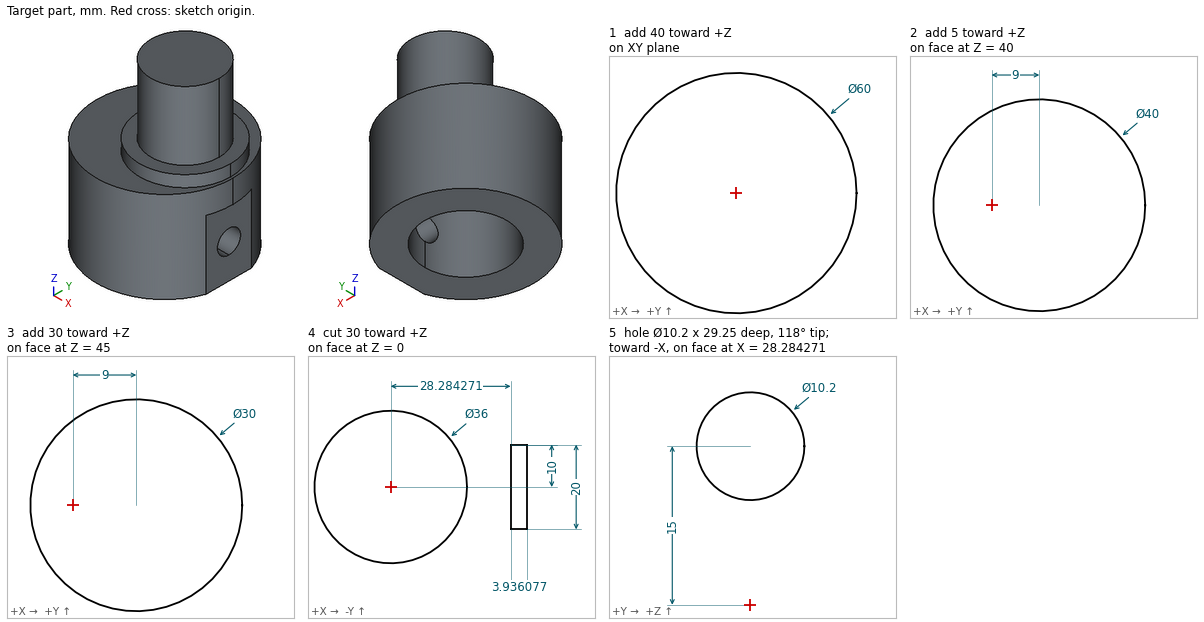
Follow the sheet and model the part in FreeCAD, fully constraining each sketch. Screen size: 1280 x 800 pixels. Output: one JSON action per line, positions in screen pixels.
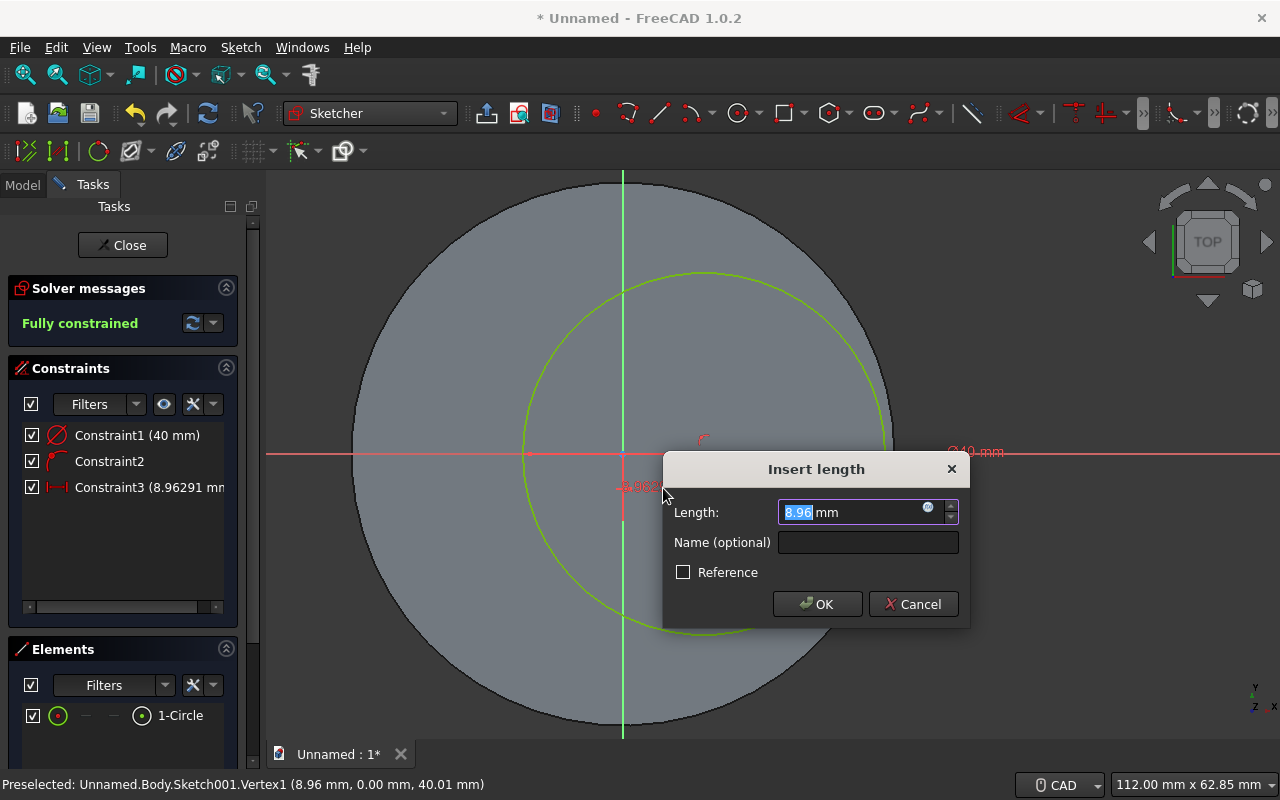
{"action": "type", "text": "9"}
{"action": "key", "text": "Return"}
{"action": "key", "text": "Escape"}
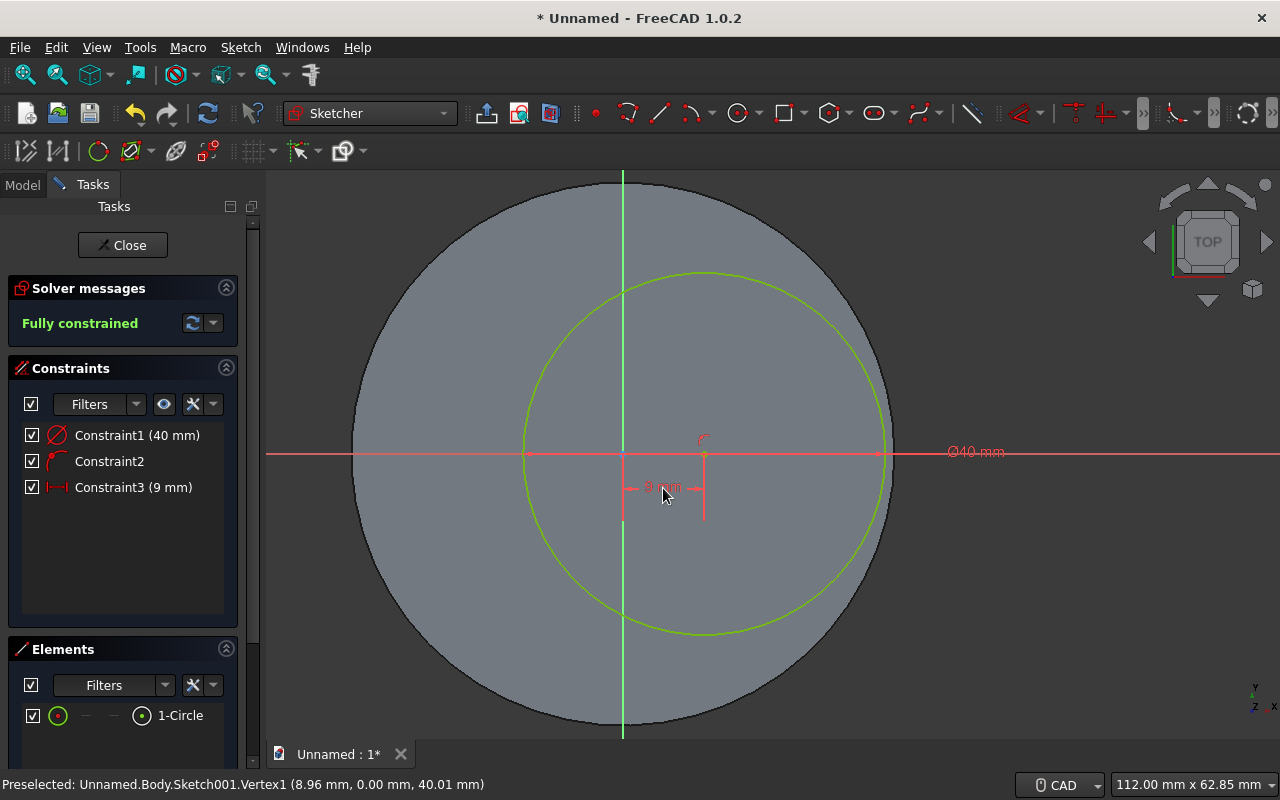
{"action": "left_click", "coordinate": [123, 245]}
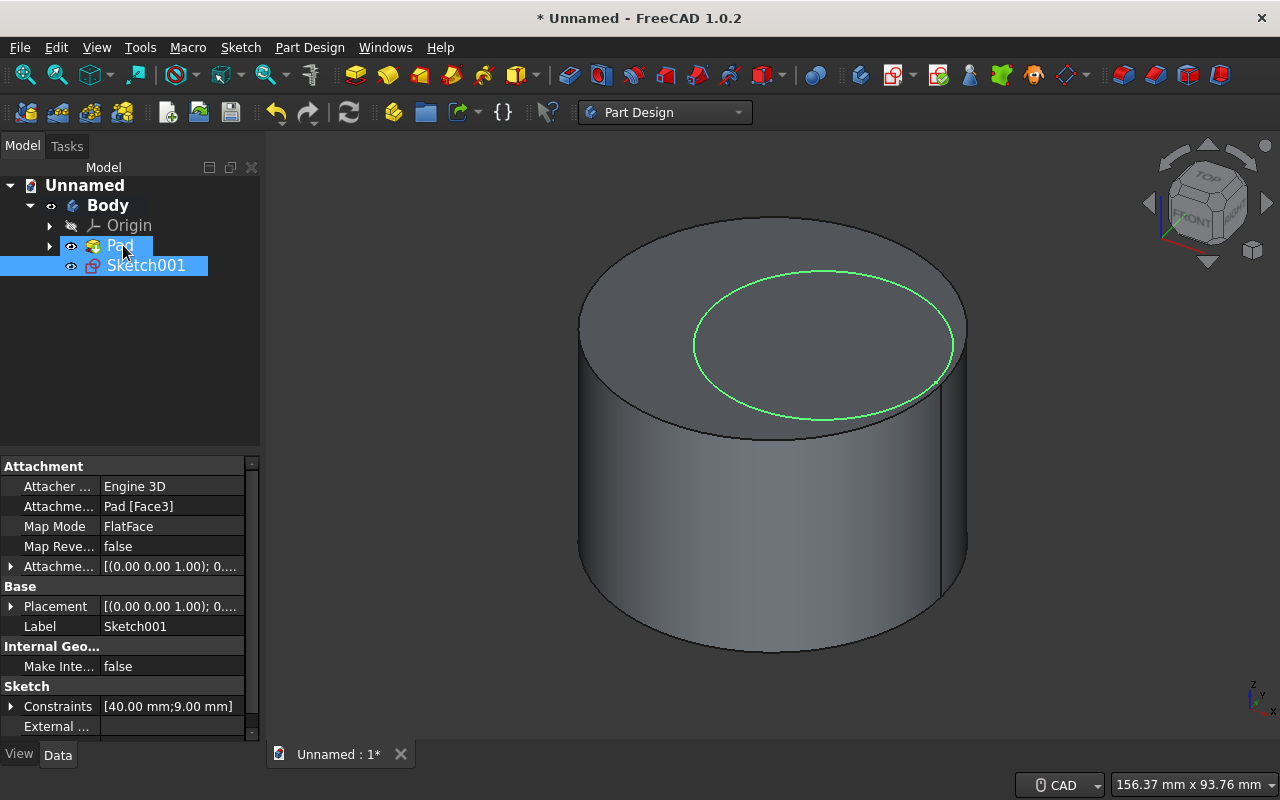
{"action": "left_click", "coordinate": [356, 76]}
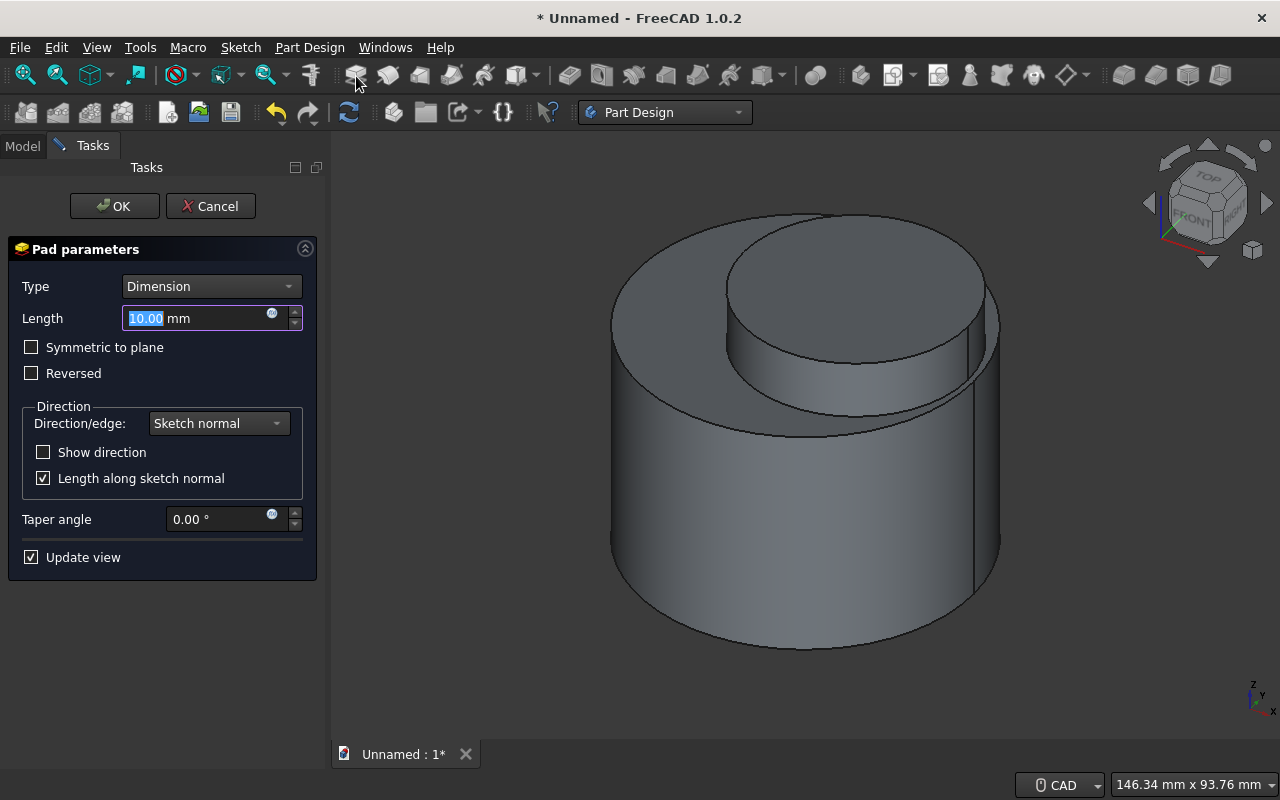
{"action": "type", "text": "5"}
{"action": "key", "text": "Tab"}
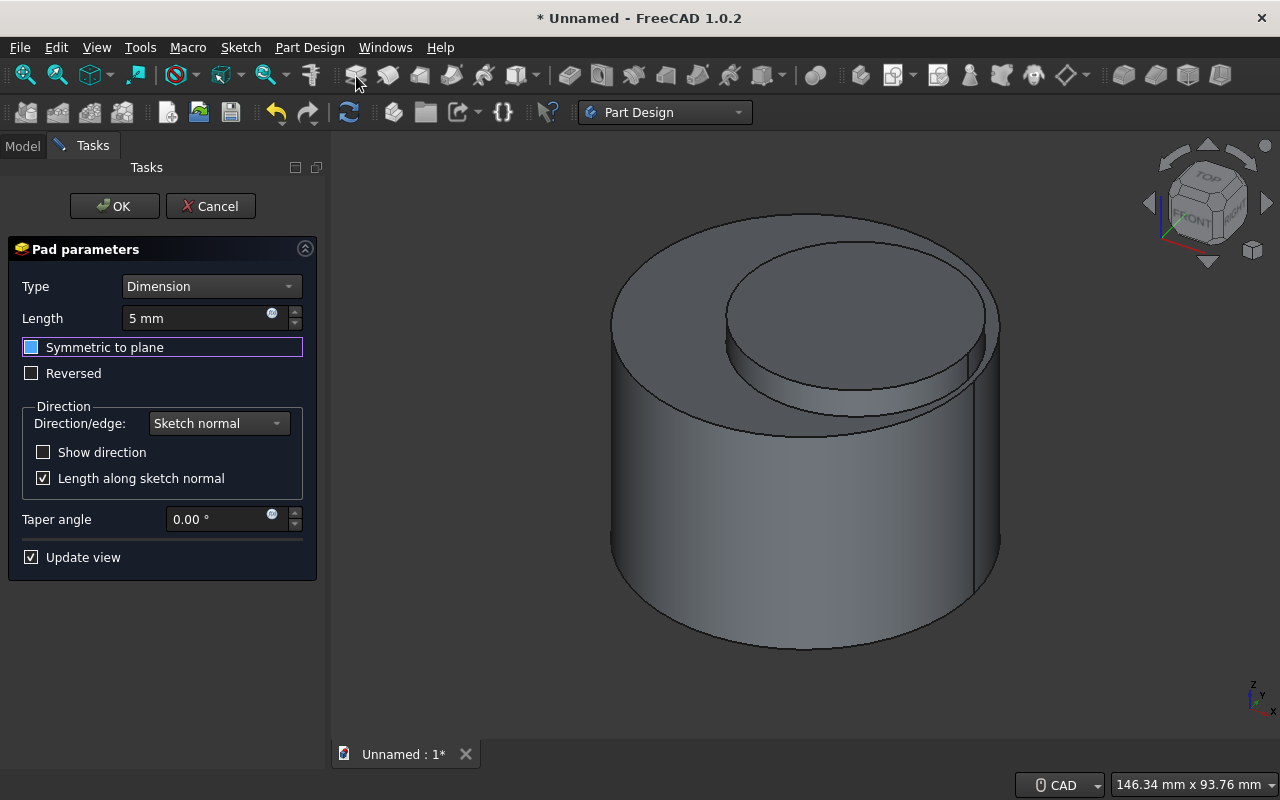
{"action": "left_click", "coordinate": [115, 206]}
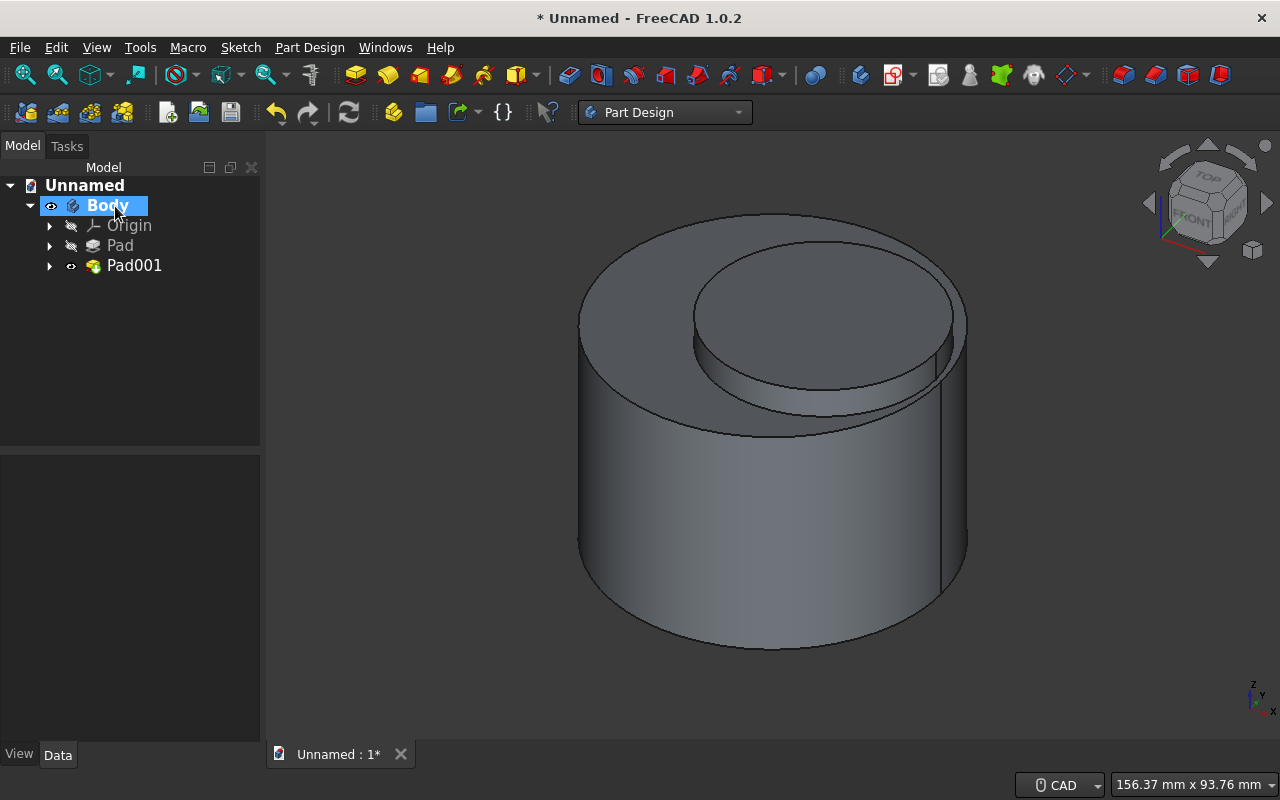
{"action": "left_click", "coordinate": [823, 315]}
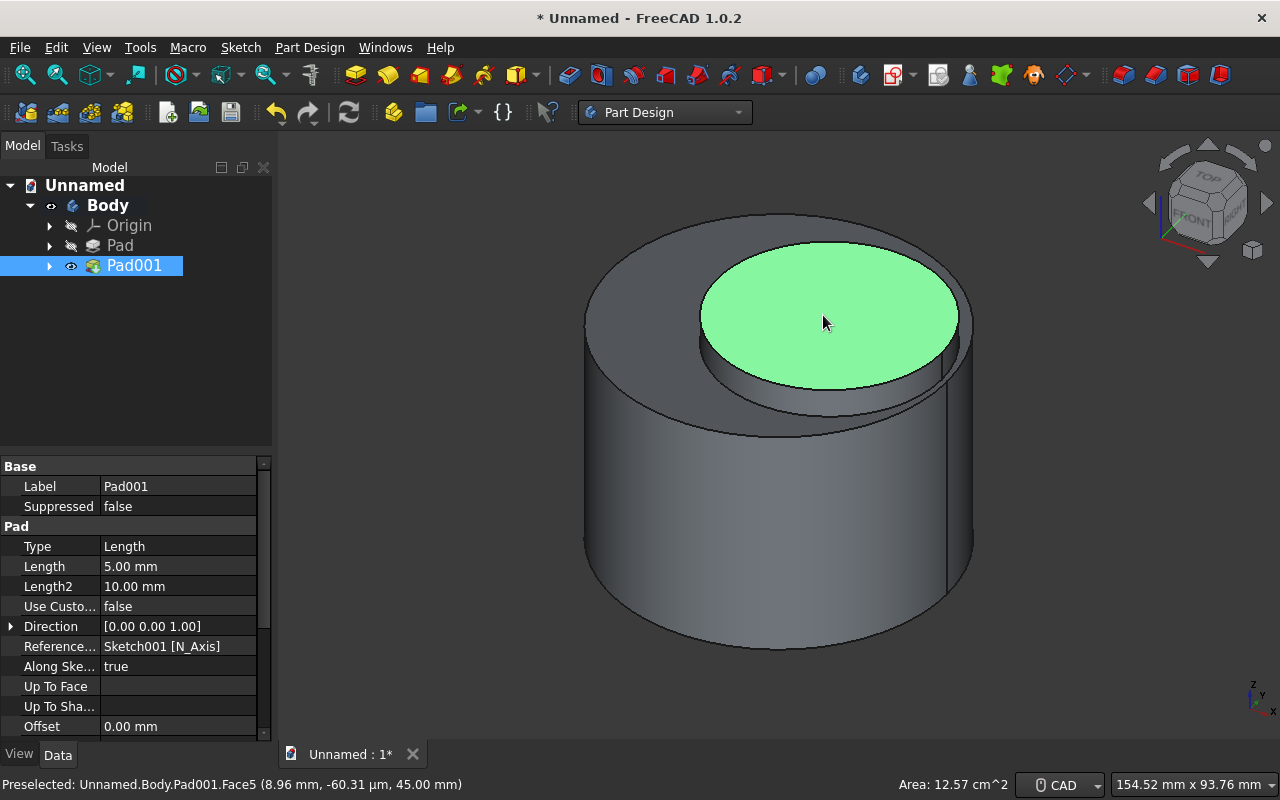
{"action": "left_click", "coordinate": [894, 76]}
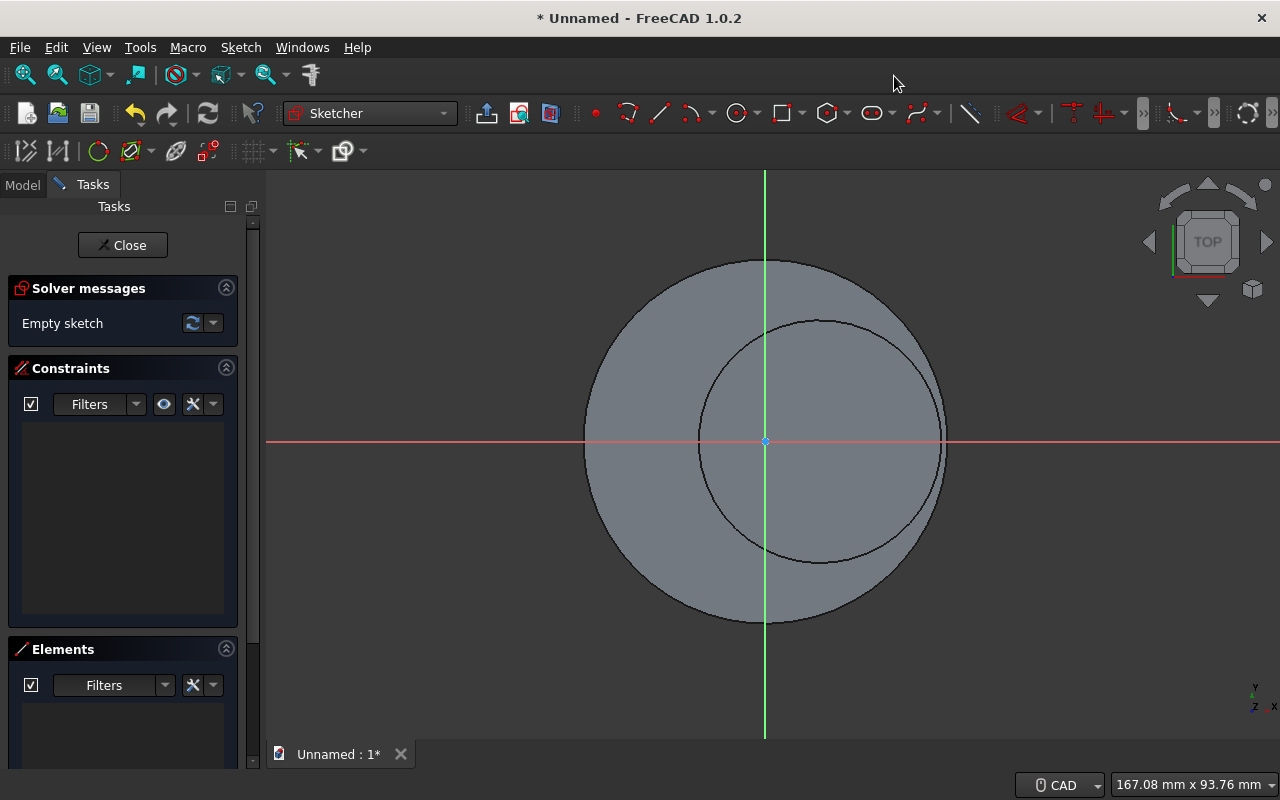
{"action": "scroll", "coordinate": [961, 426], "scroll_direction": "up", "scroll_amount": 3}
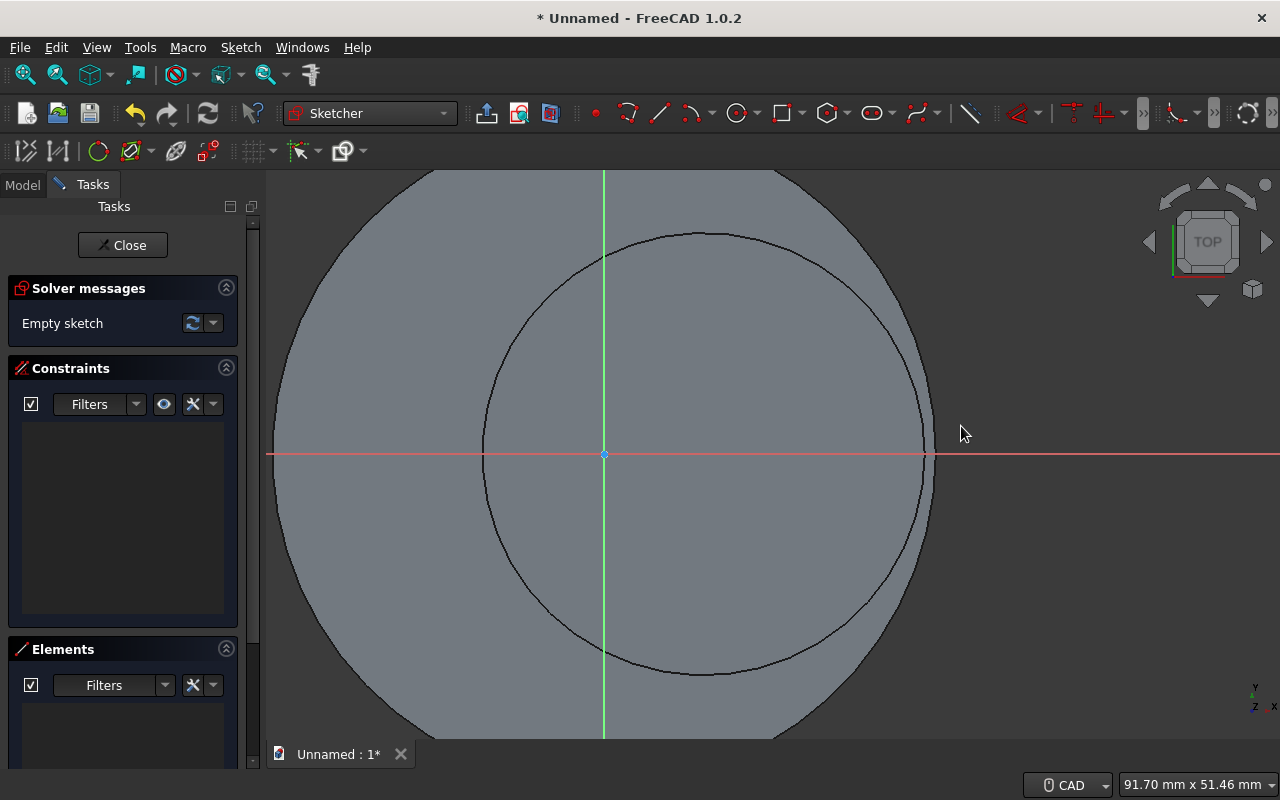
{"action": "key", "text": "g c"}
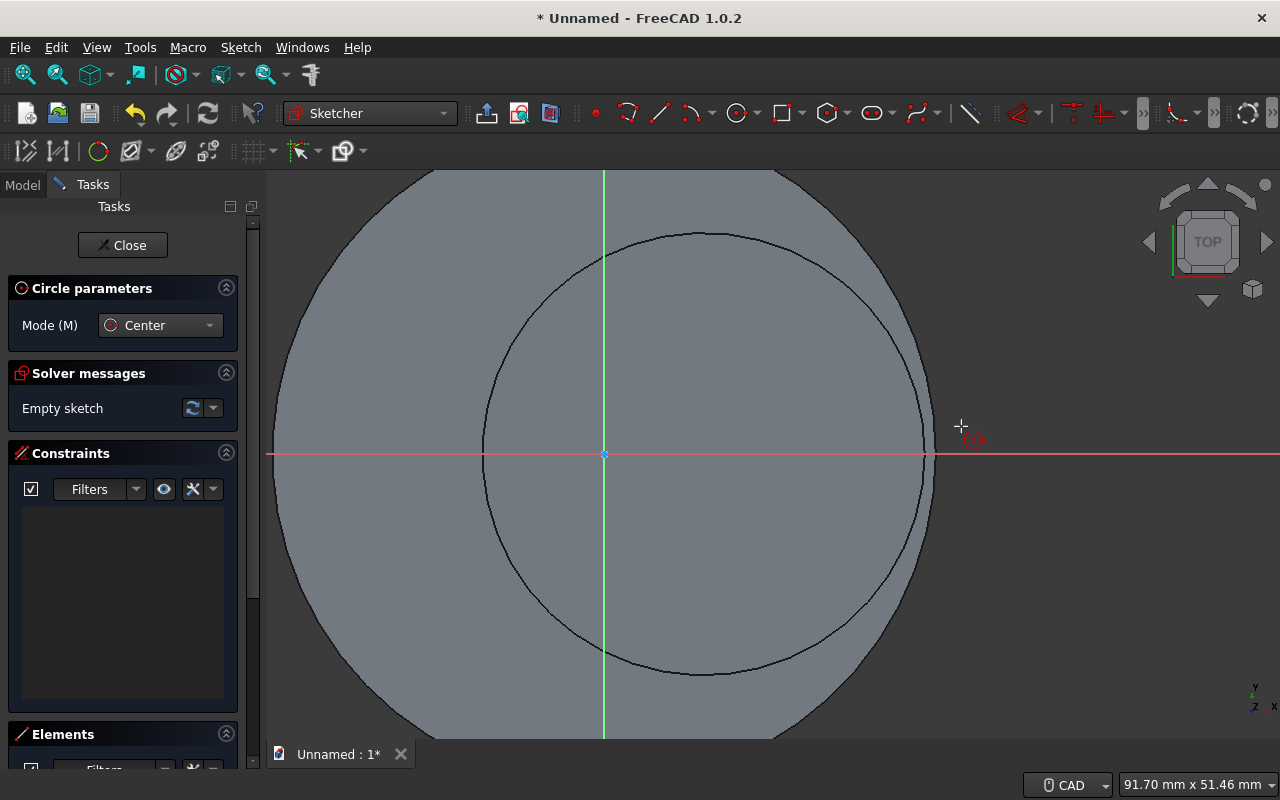
{"action": "left_click", "coordinate": [704, 454]}
{"action": "mouse_move", "coordinate": [821, 337]}